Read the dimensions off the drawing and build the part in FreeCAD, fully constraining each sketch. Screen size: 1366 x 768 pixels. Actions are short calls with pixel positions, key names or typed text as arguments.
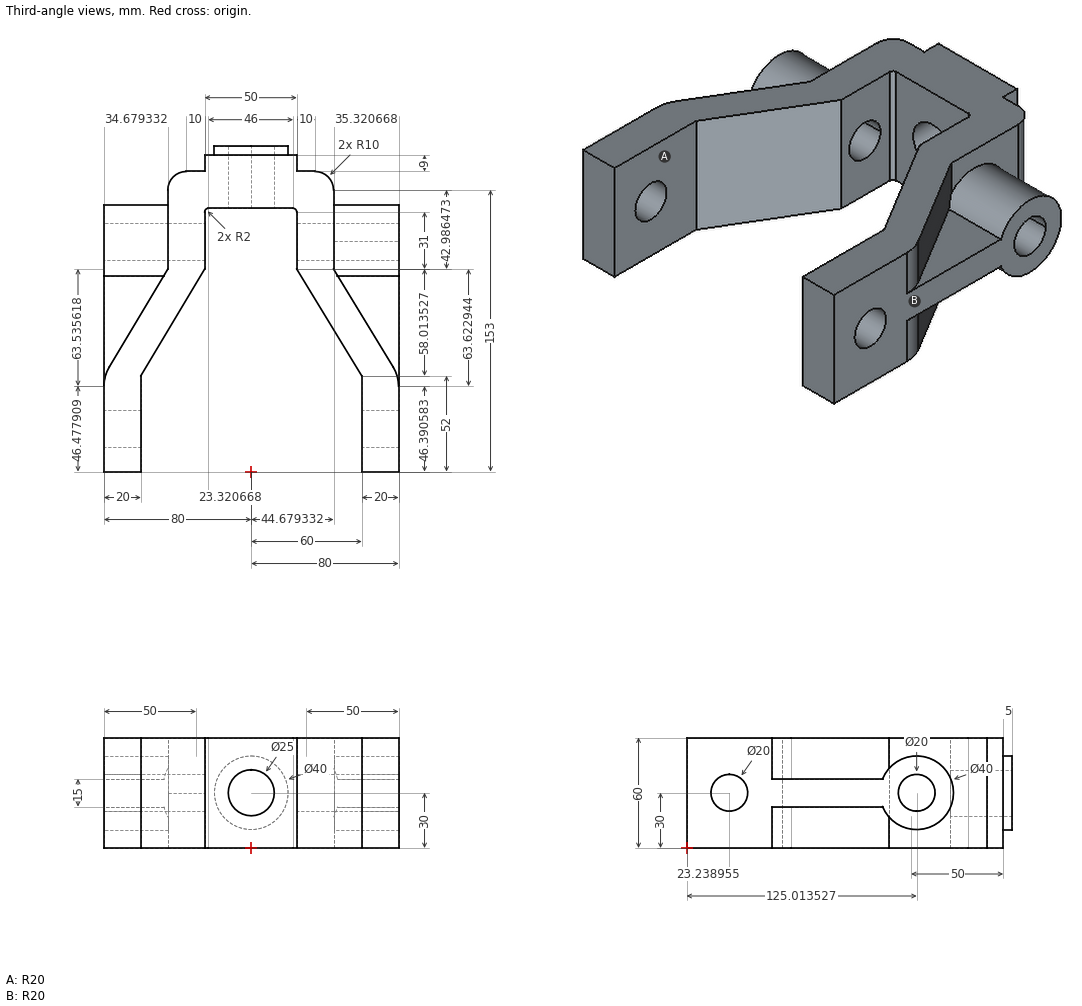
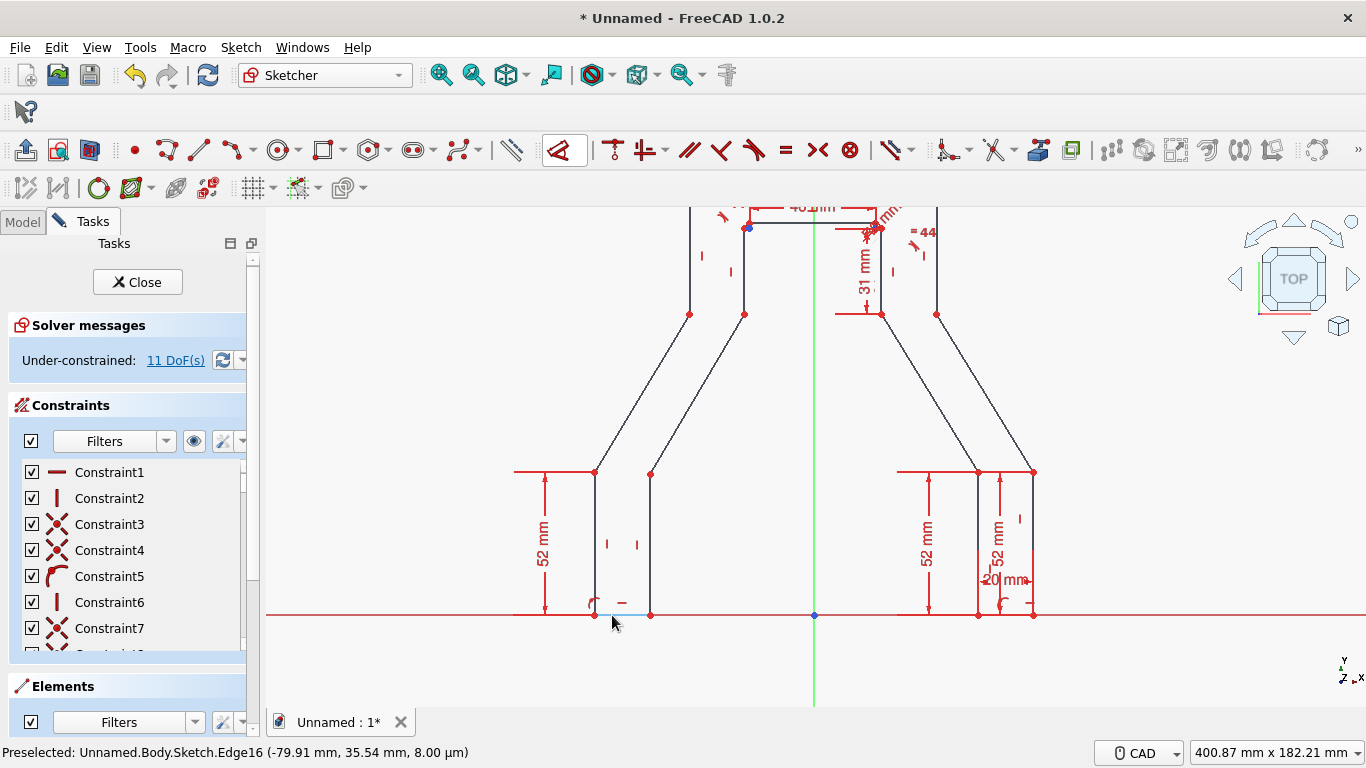
click(611, 615)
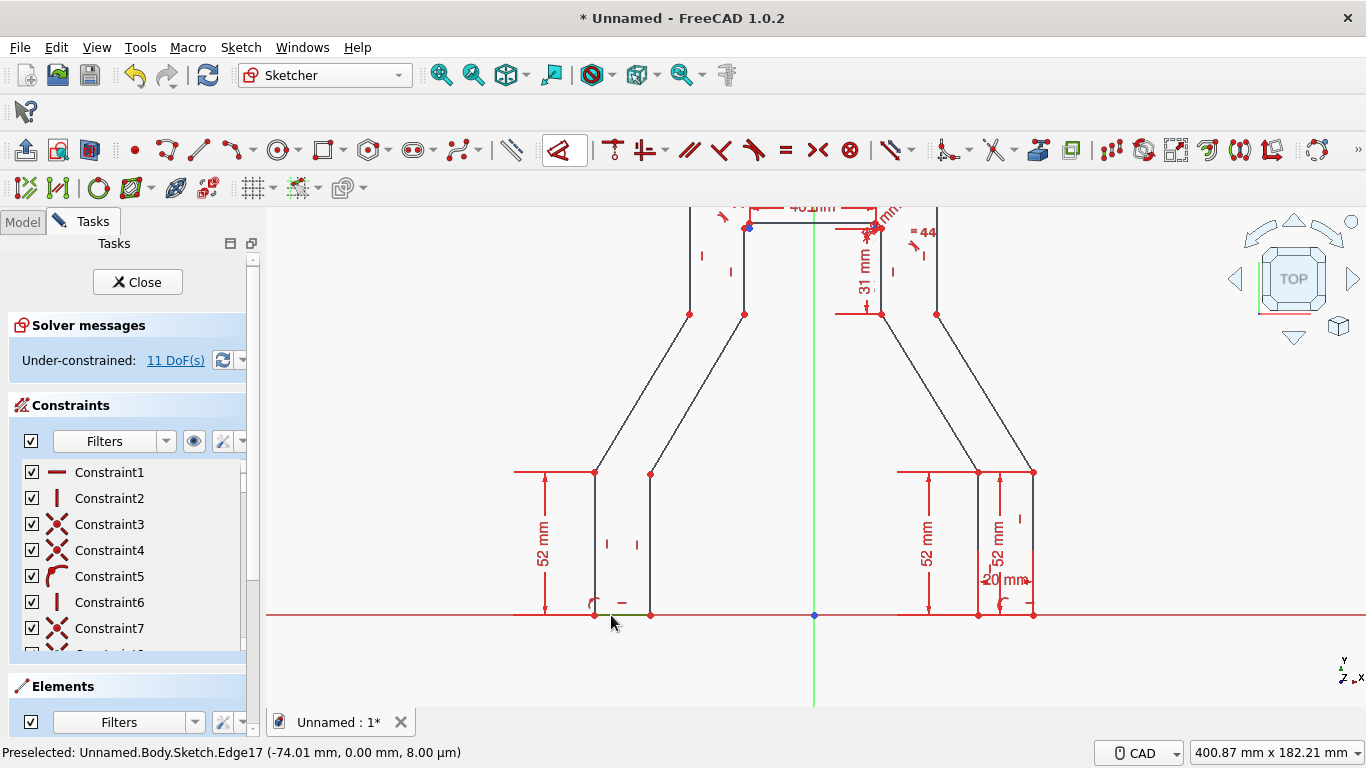
key(l)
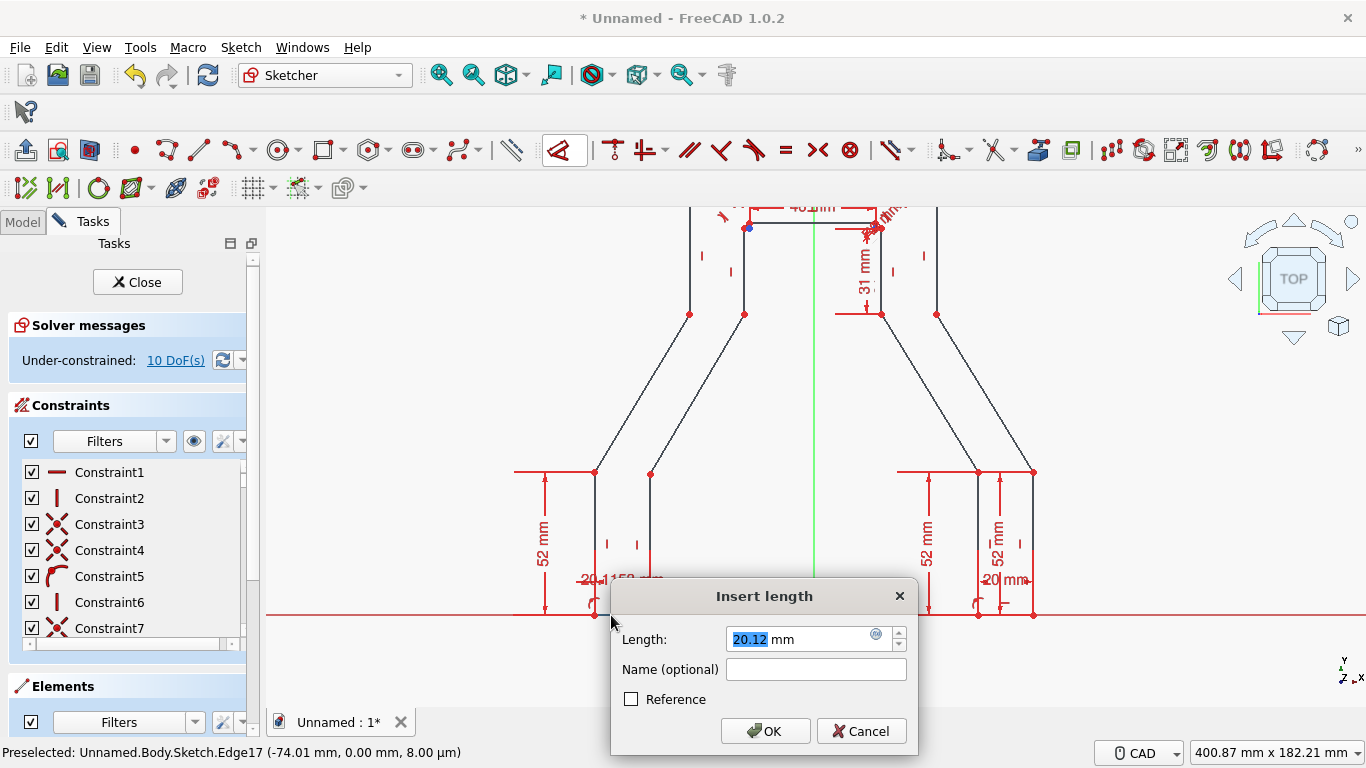
text(20)
key(Return)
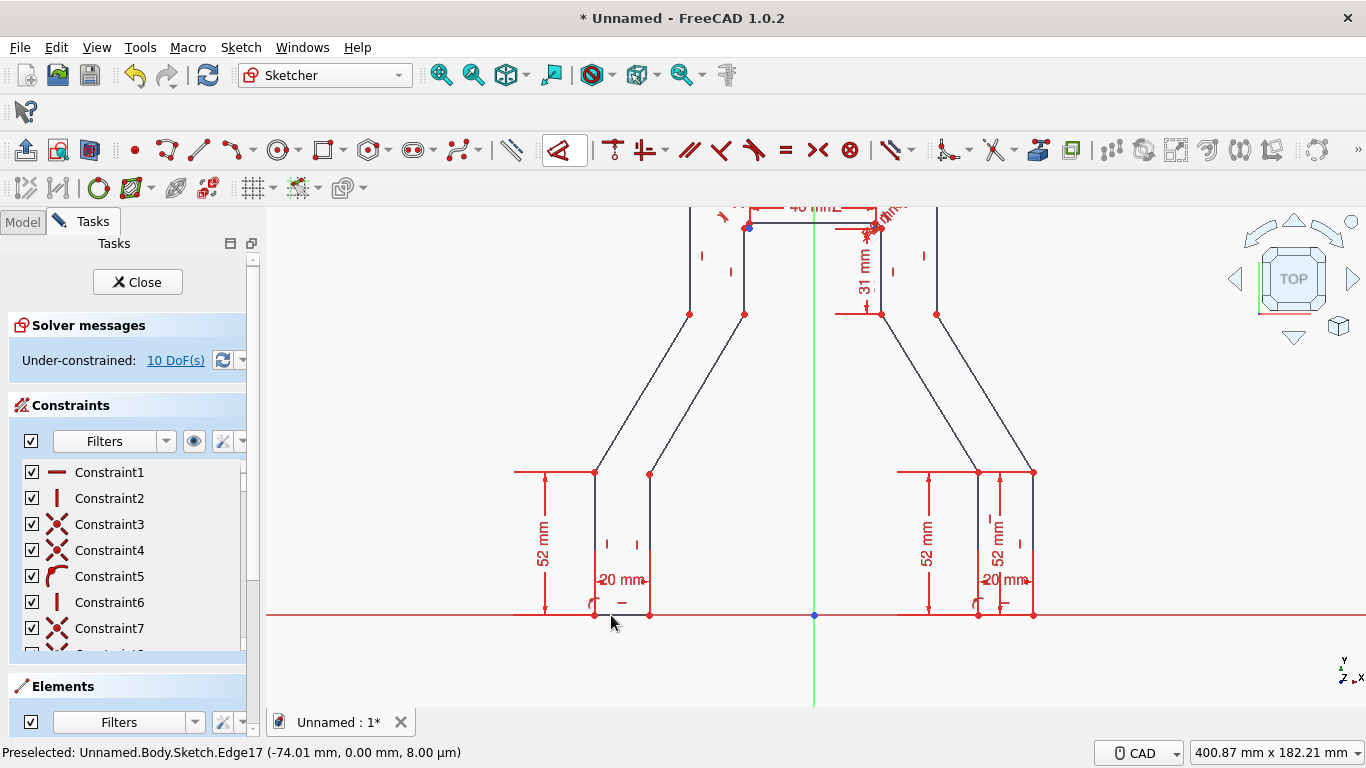
click(650, 573)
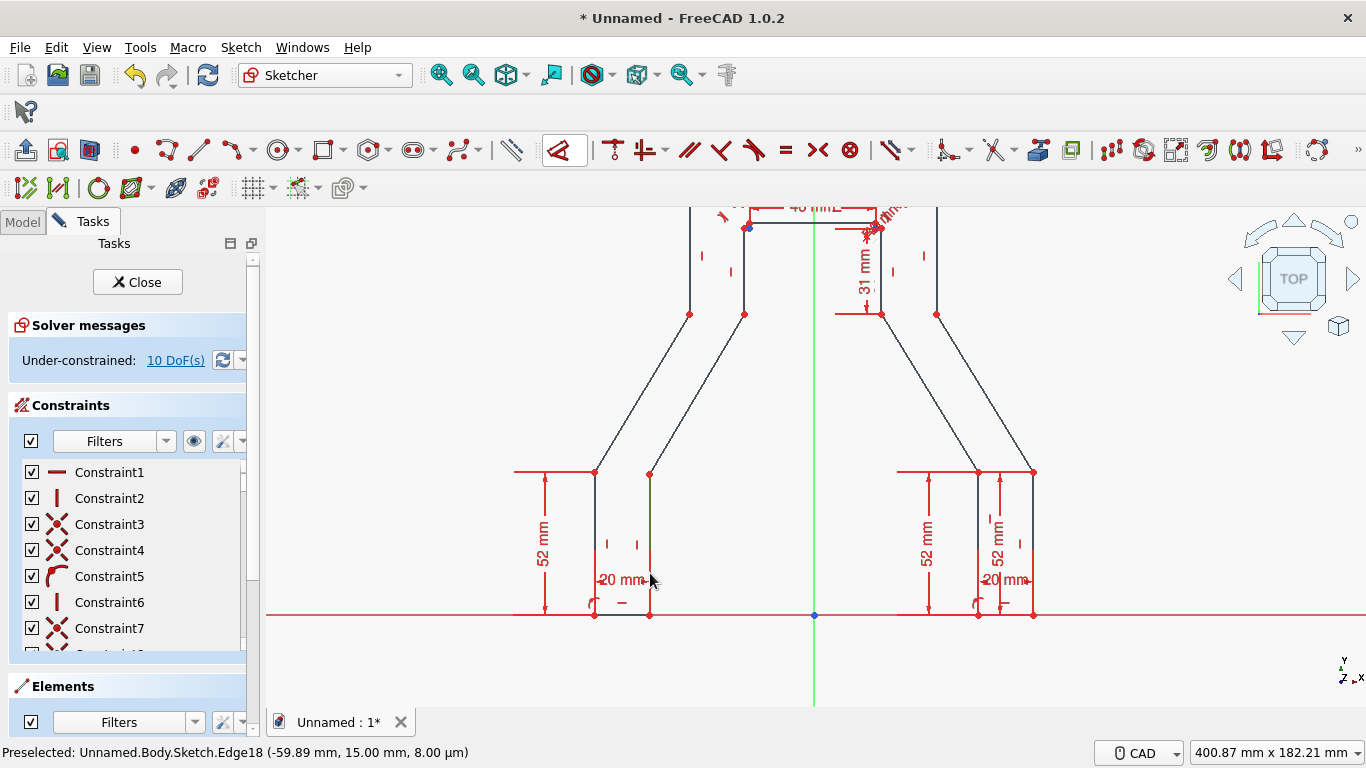
key(i)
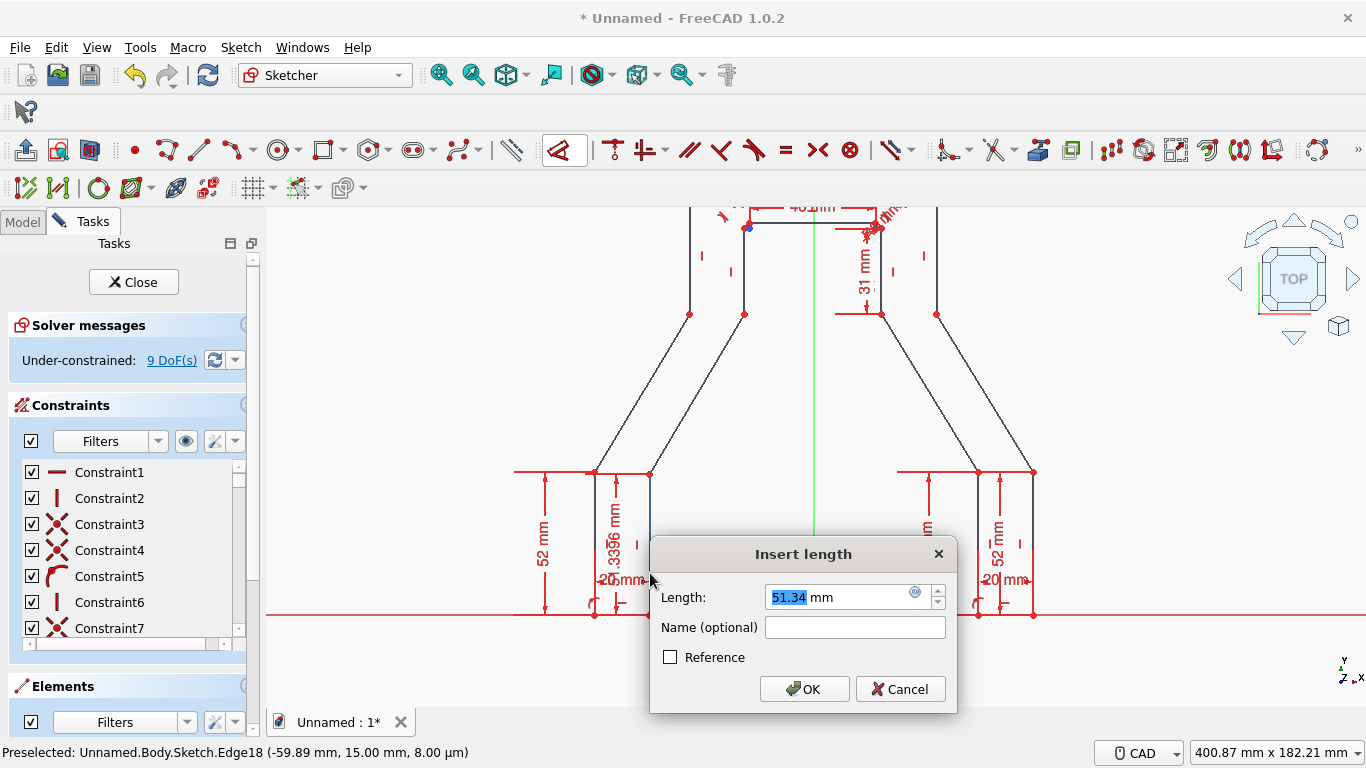
text(52)
key(Return)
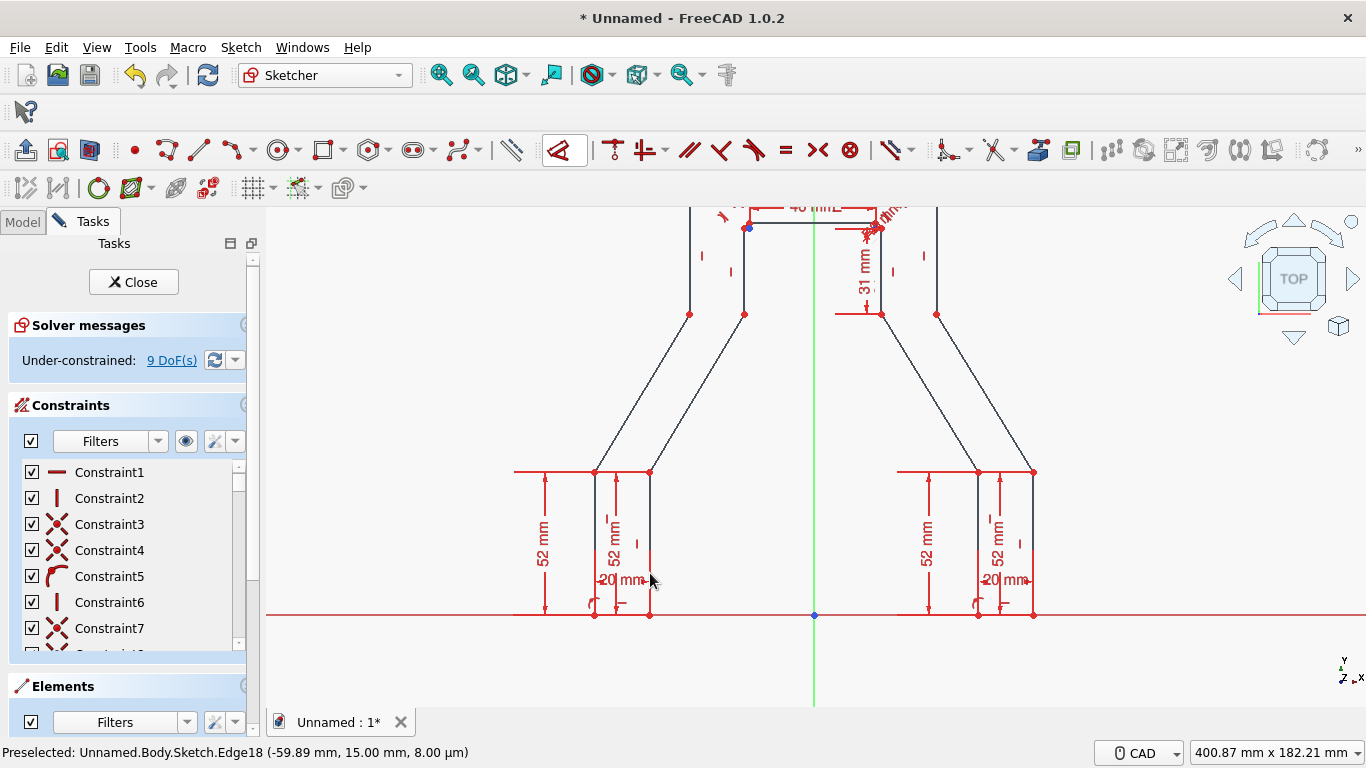
click(744, 289)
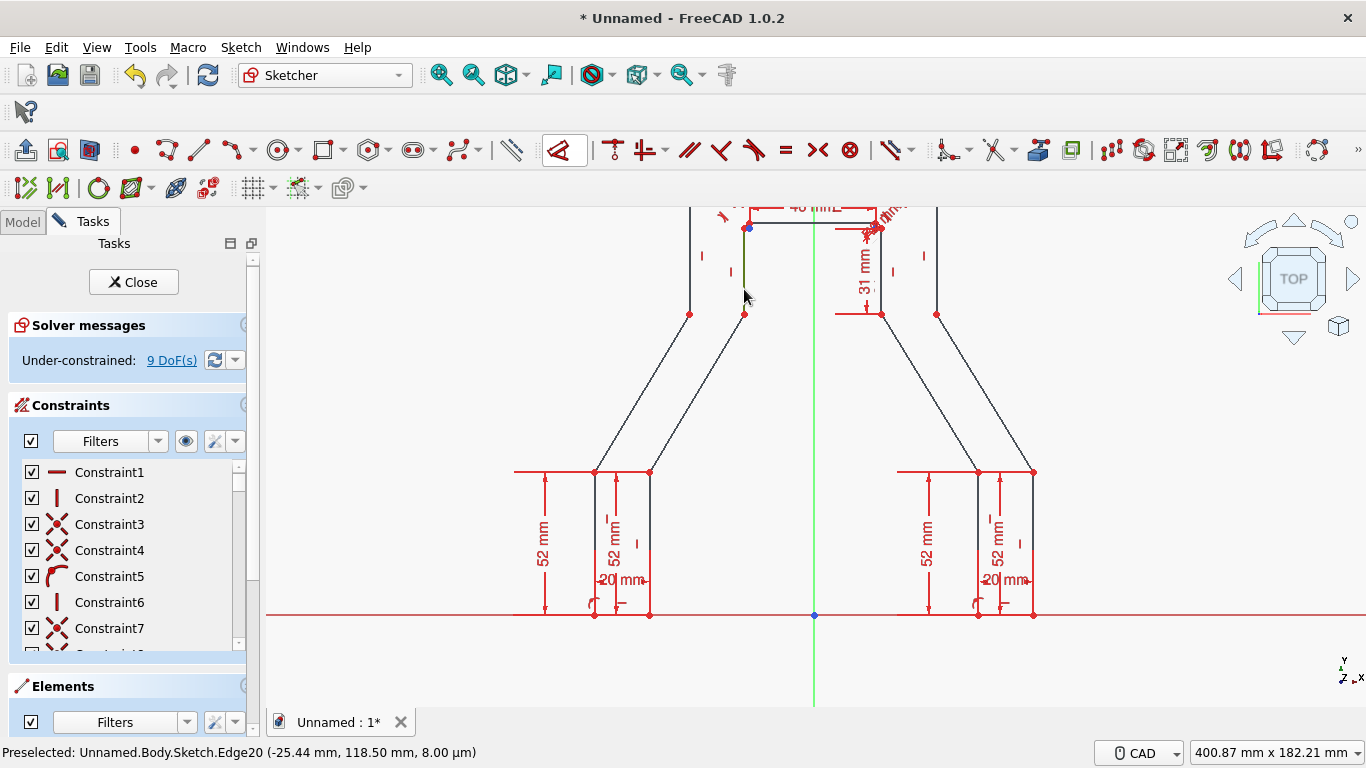
key(i)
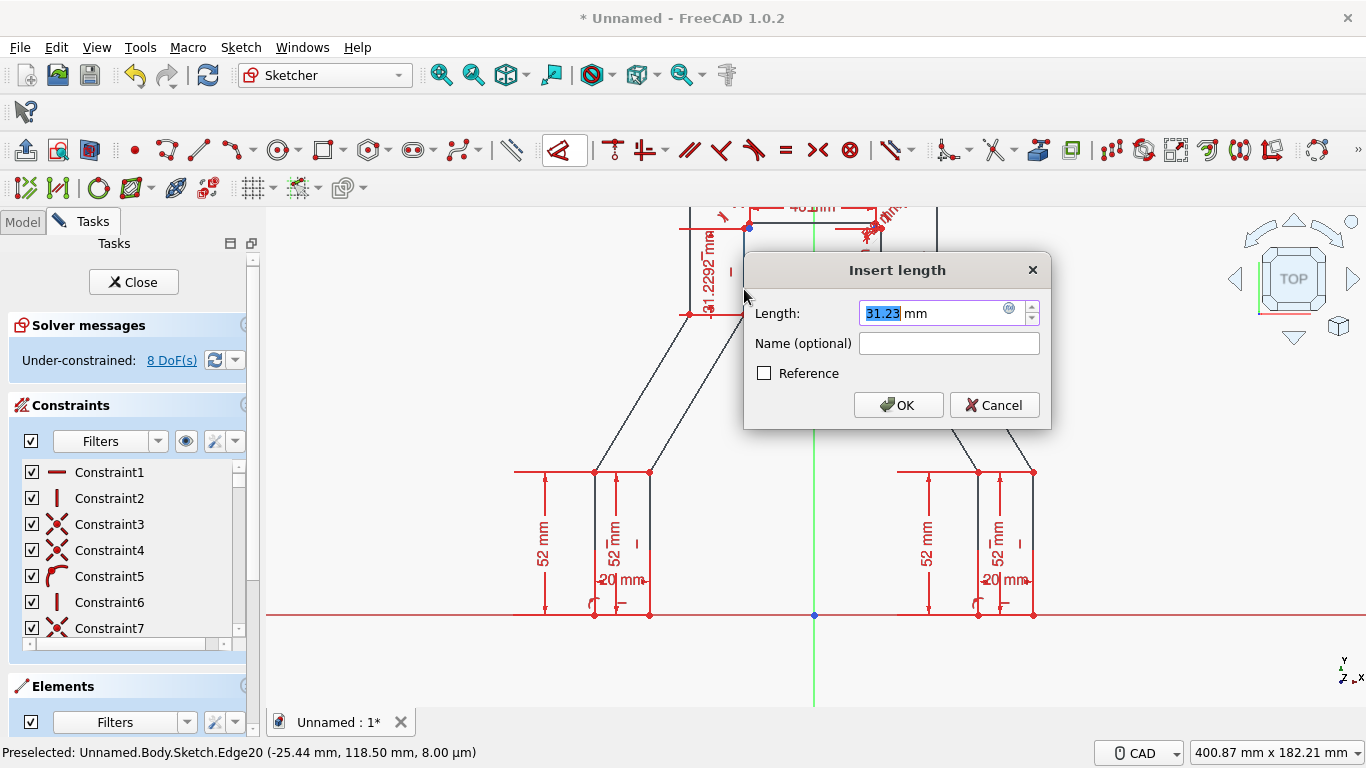
text(31)
key(Return)